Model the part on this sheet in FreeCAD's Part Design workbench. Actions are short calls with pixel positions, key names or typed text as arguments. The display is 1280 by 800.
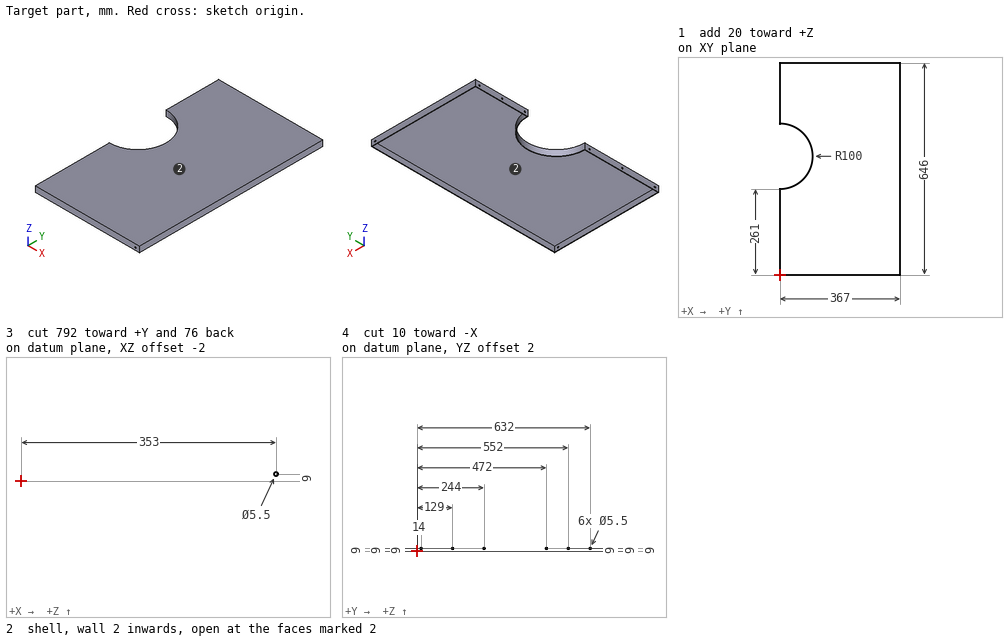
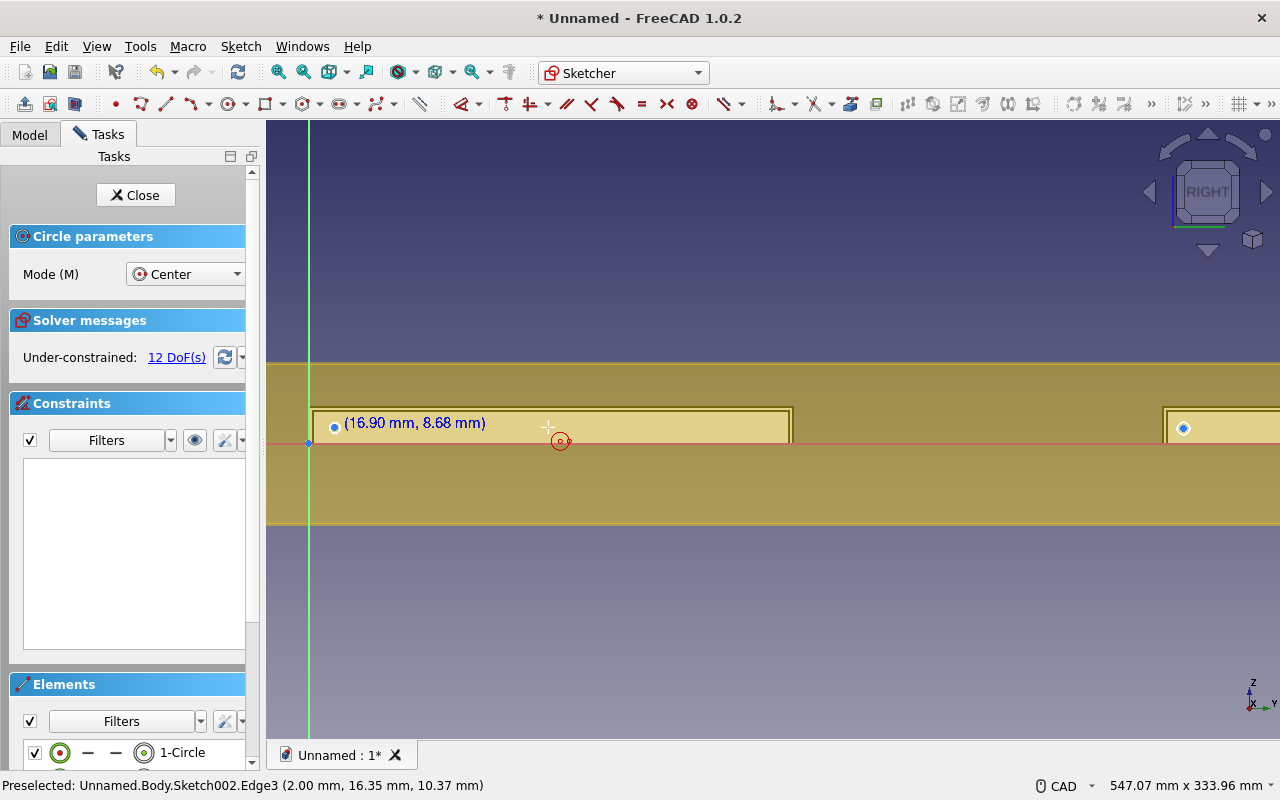
click(548, 427)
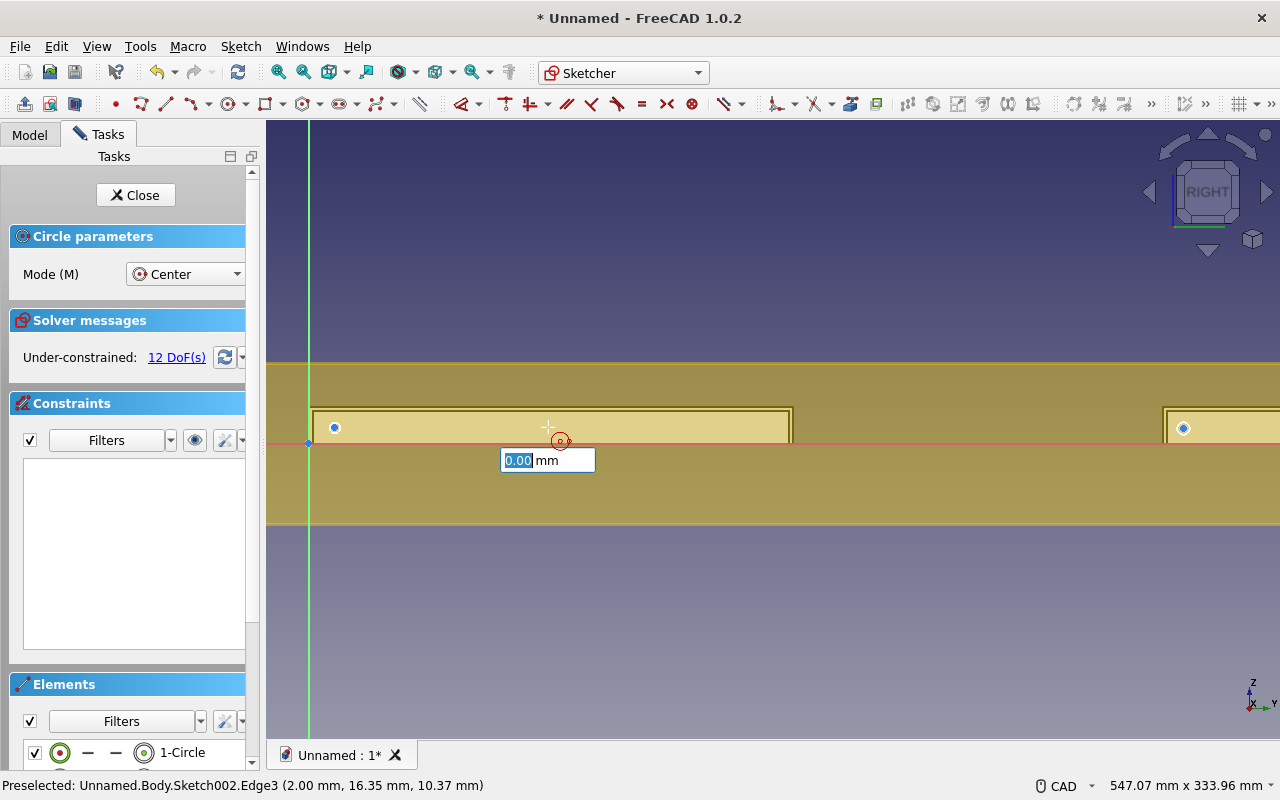
scroll(552, 424, up, 6)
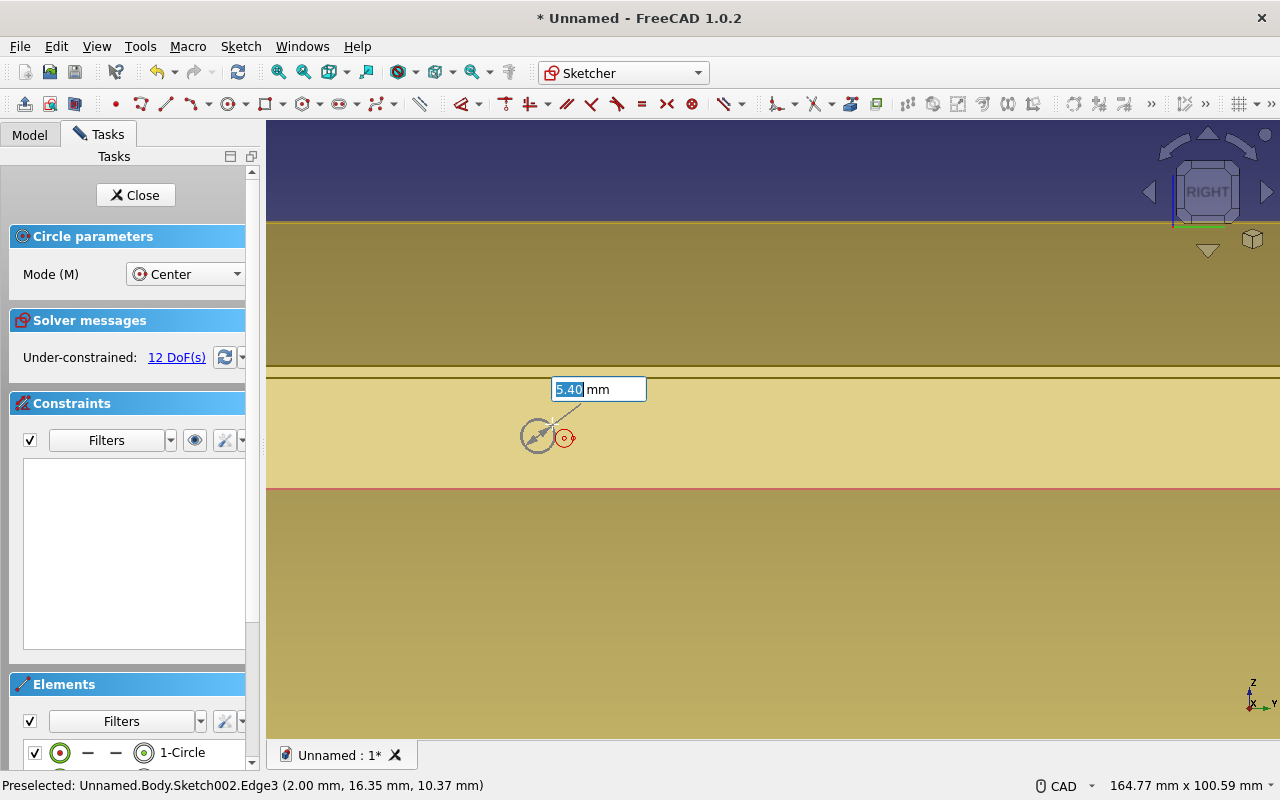
click(550, 422)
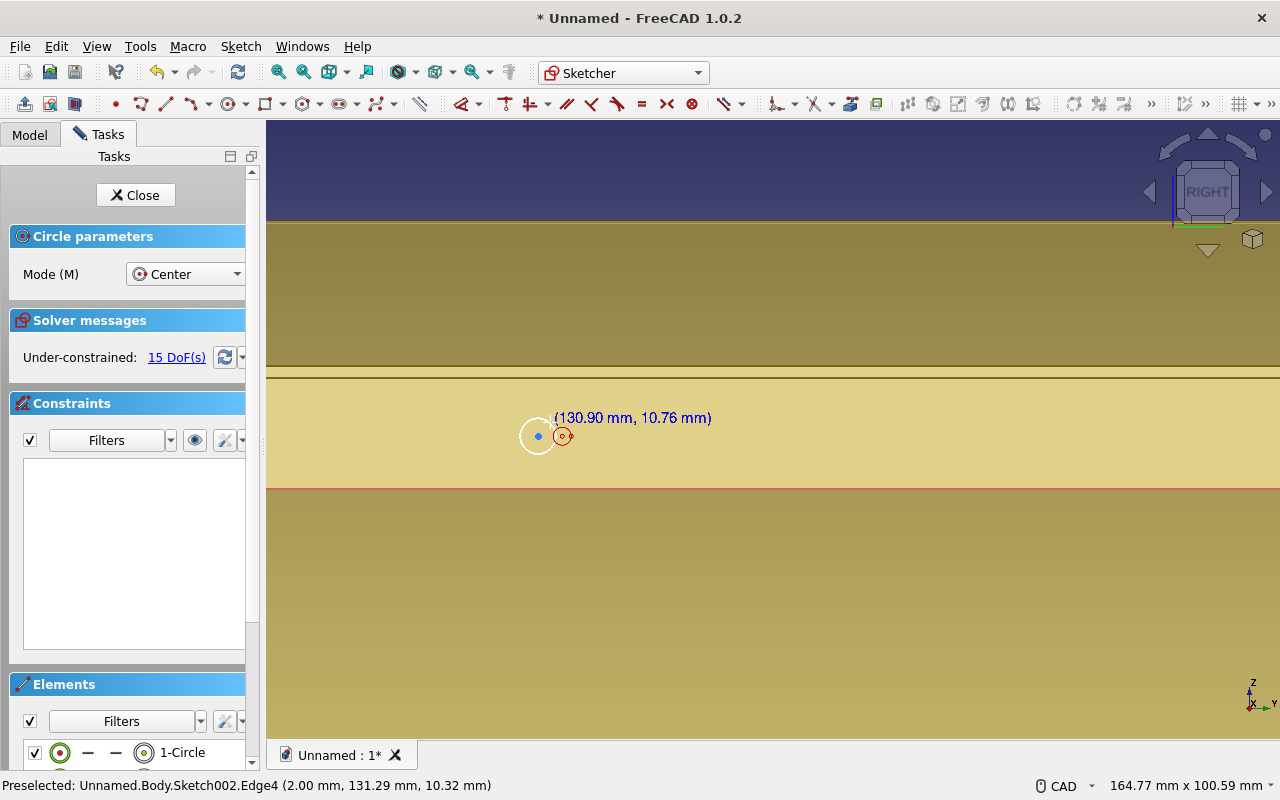
scroll(549, 426, down, 10)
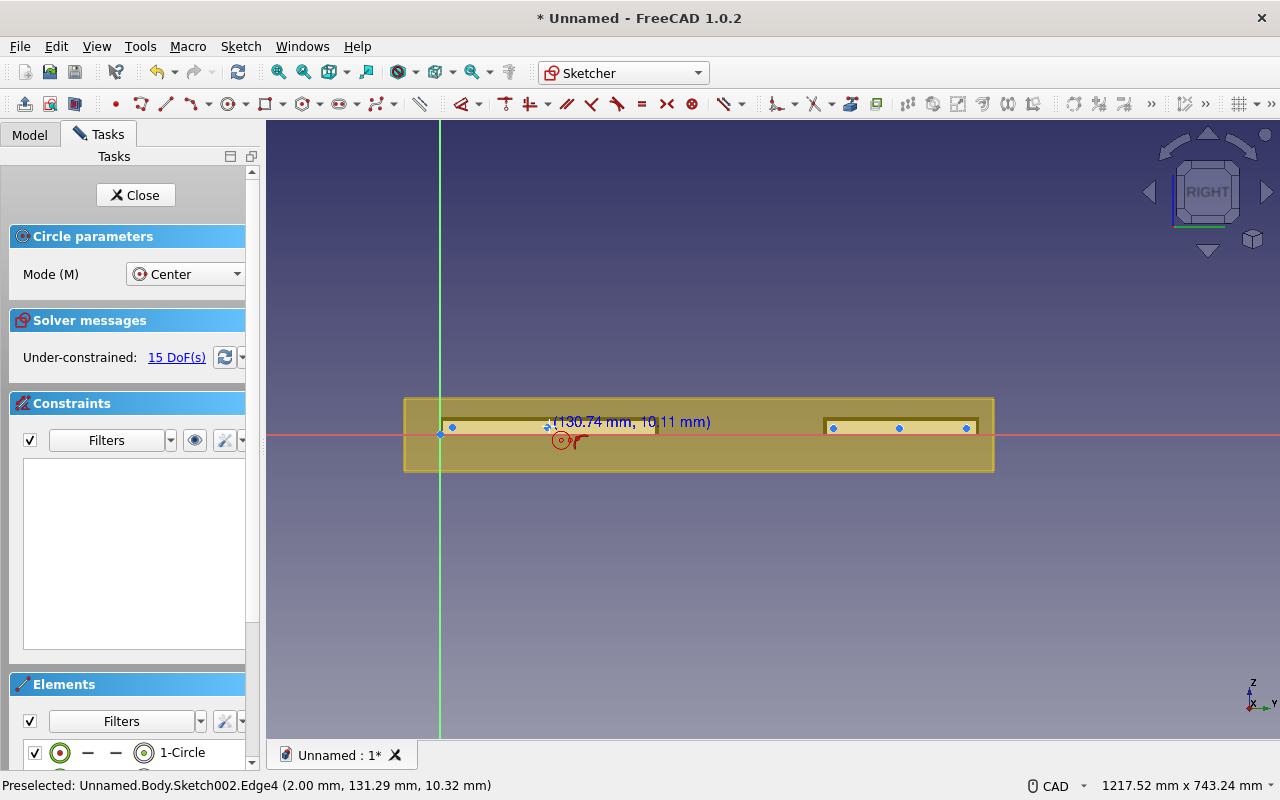
scroll(644, 427, up, 12)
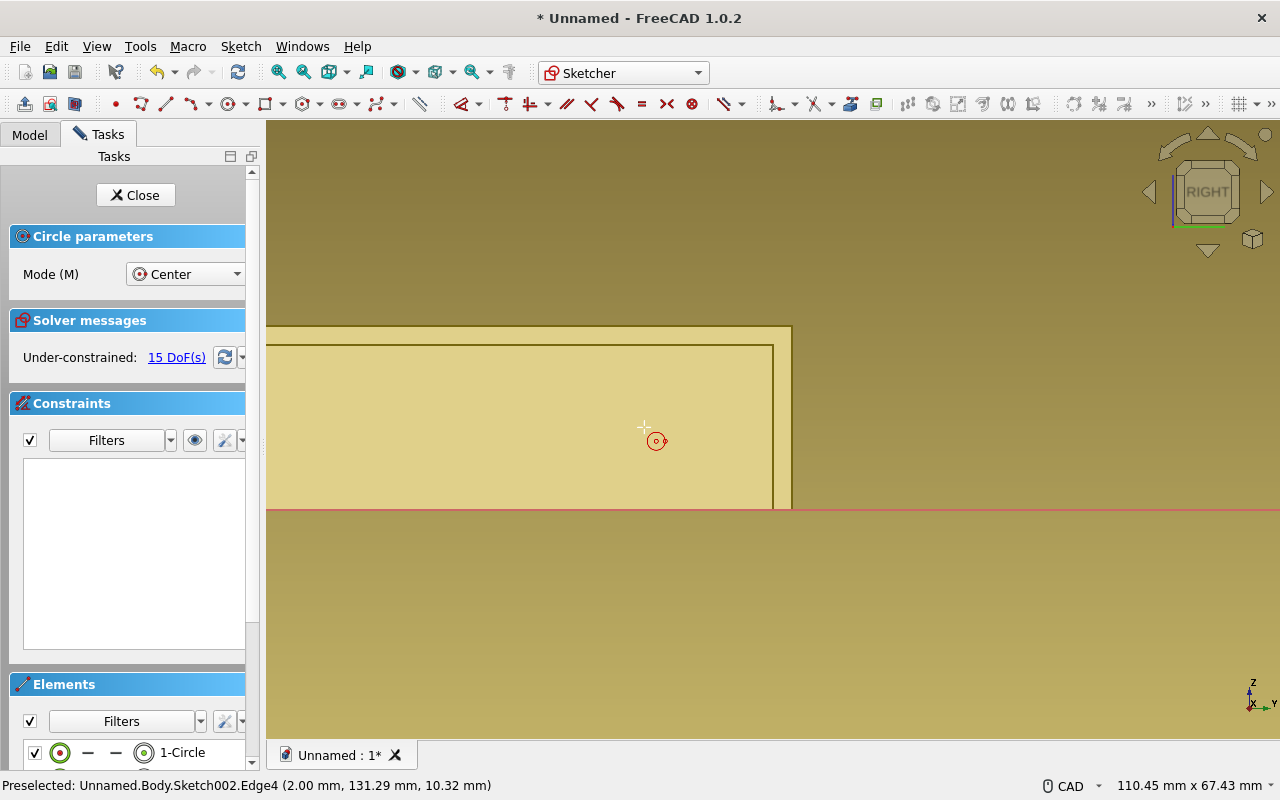
scroll(644, 427, down, 12)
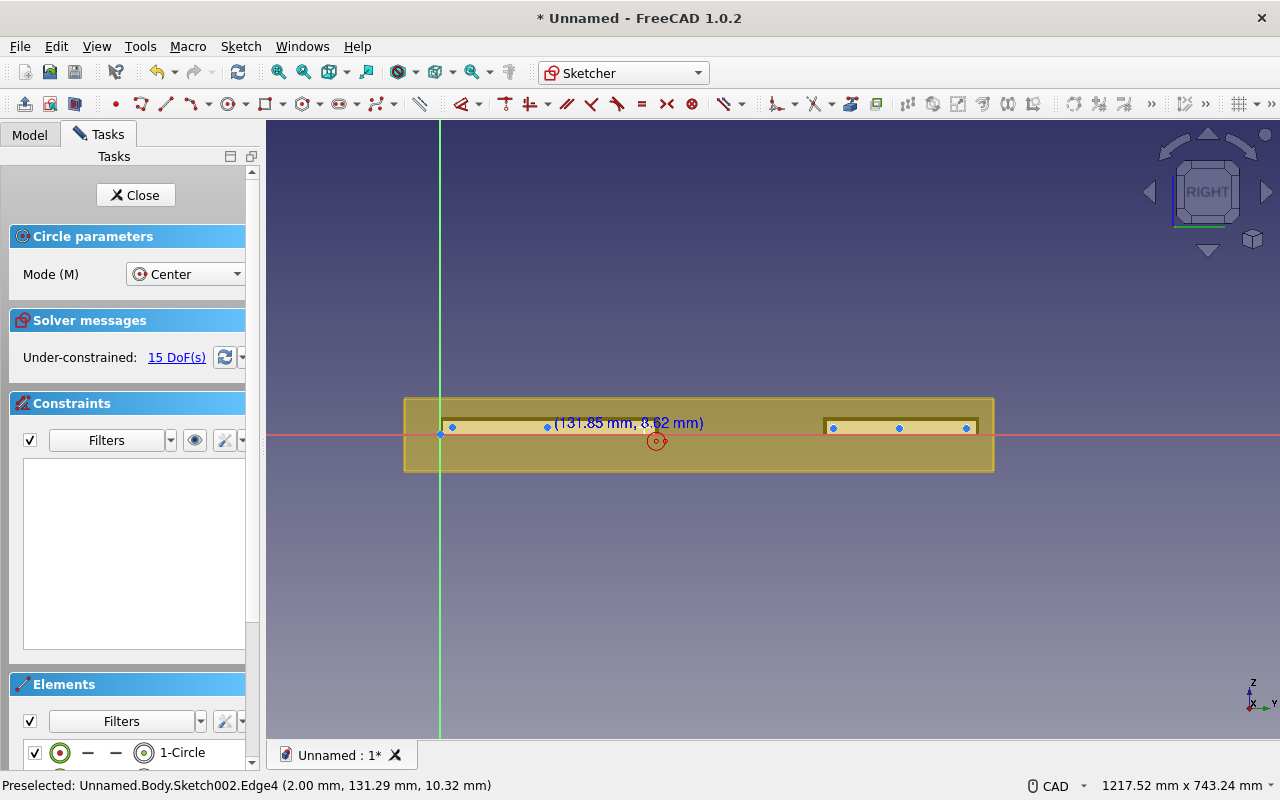
scroll(644, 427, up, 4)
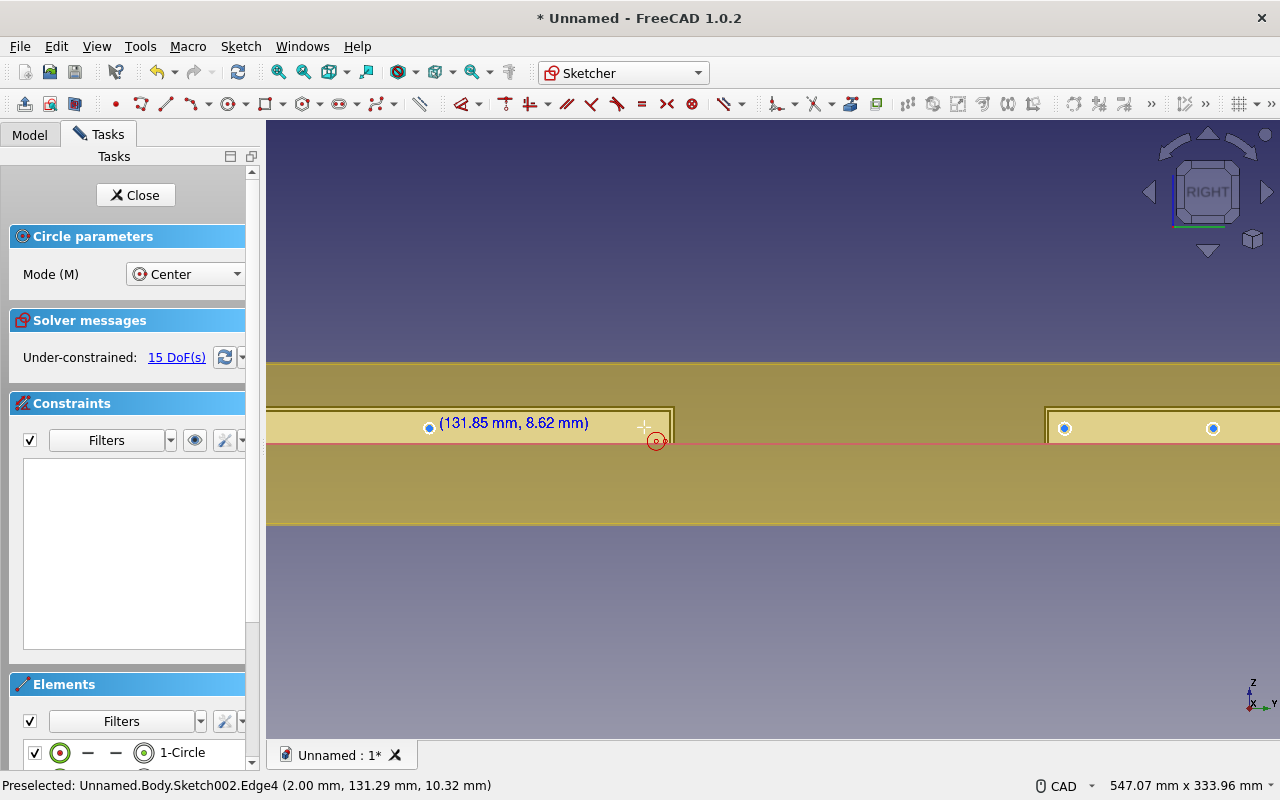
click(643, 427)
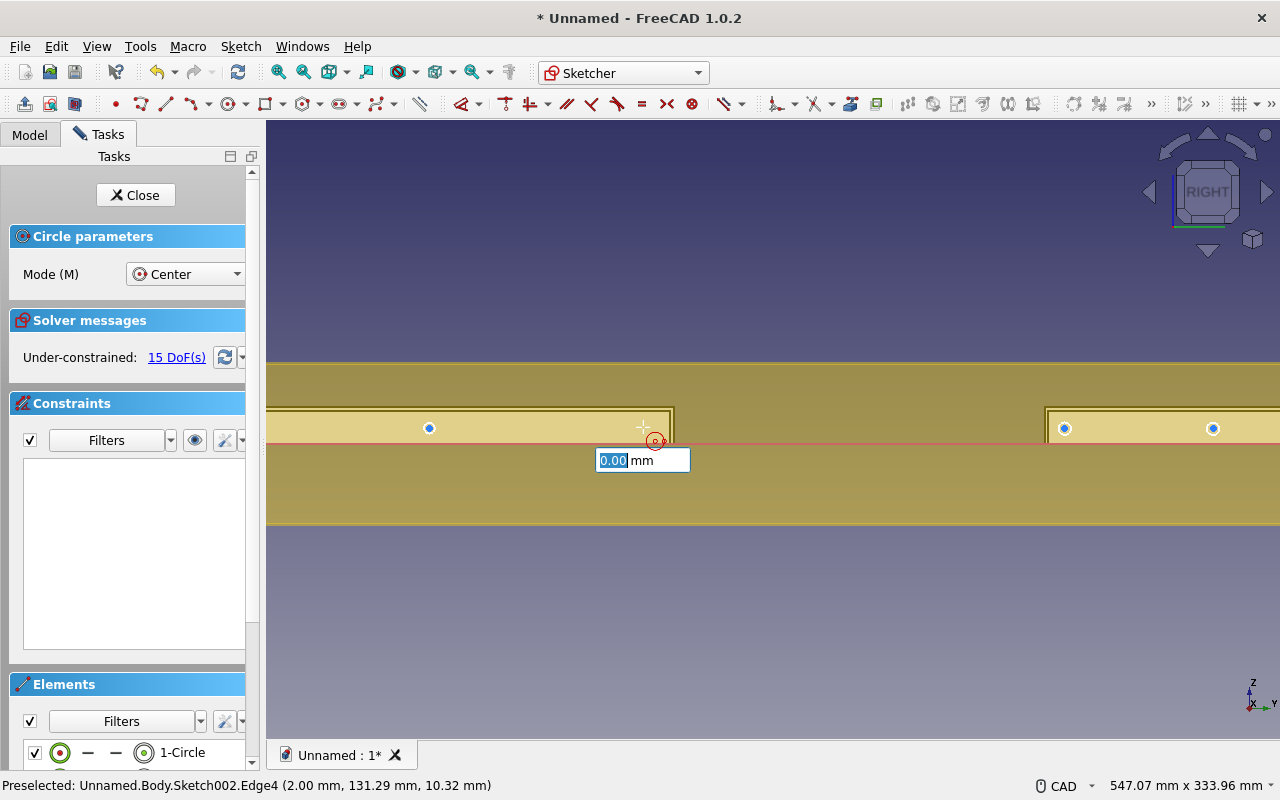
scroll(646, 424, up, 6)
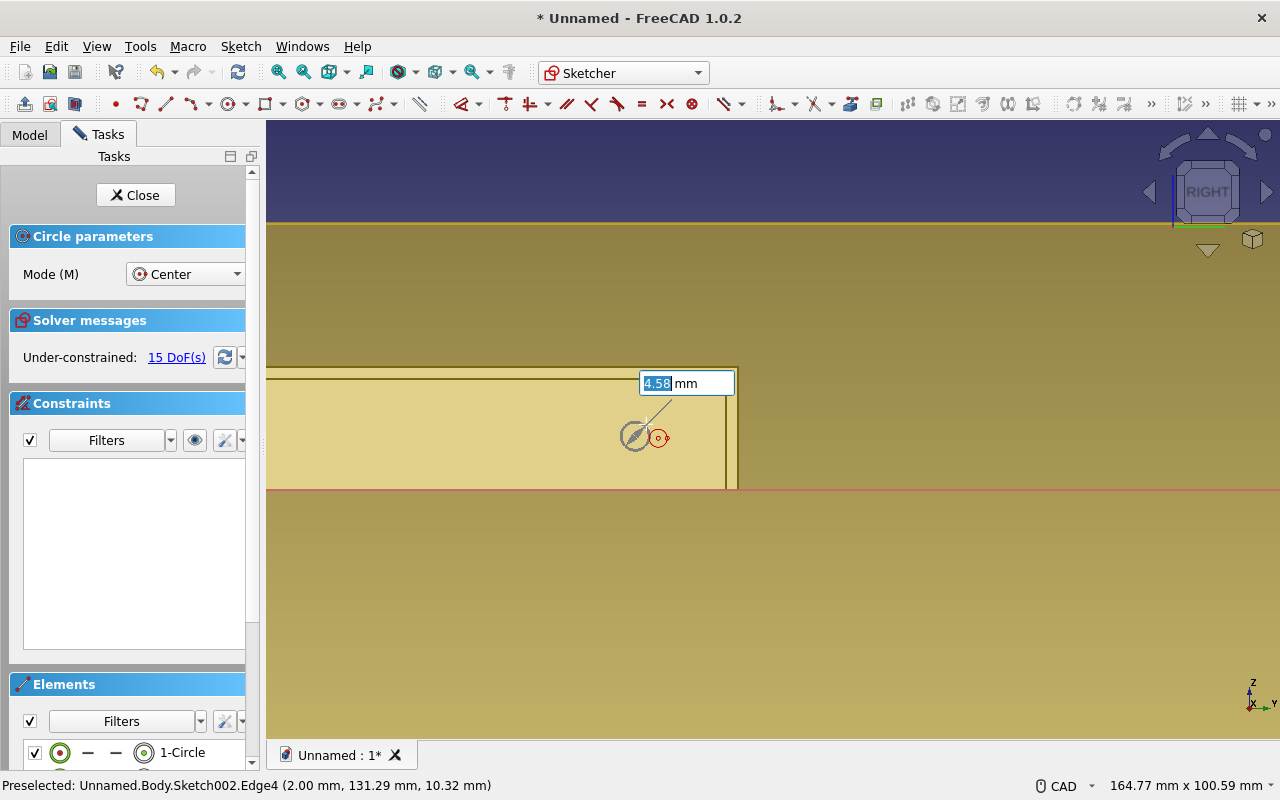
click(646, 422)
key(Escape)